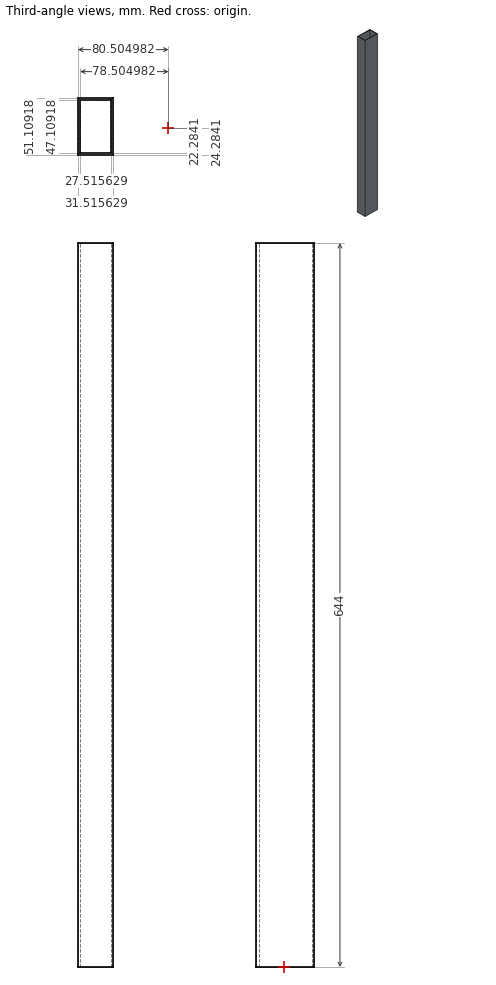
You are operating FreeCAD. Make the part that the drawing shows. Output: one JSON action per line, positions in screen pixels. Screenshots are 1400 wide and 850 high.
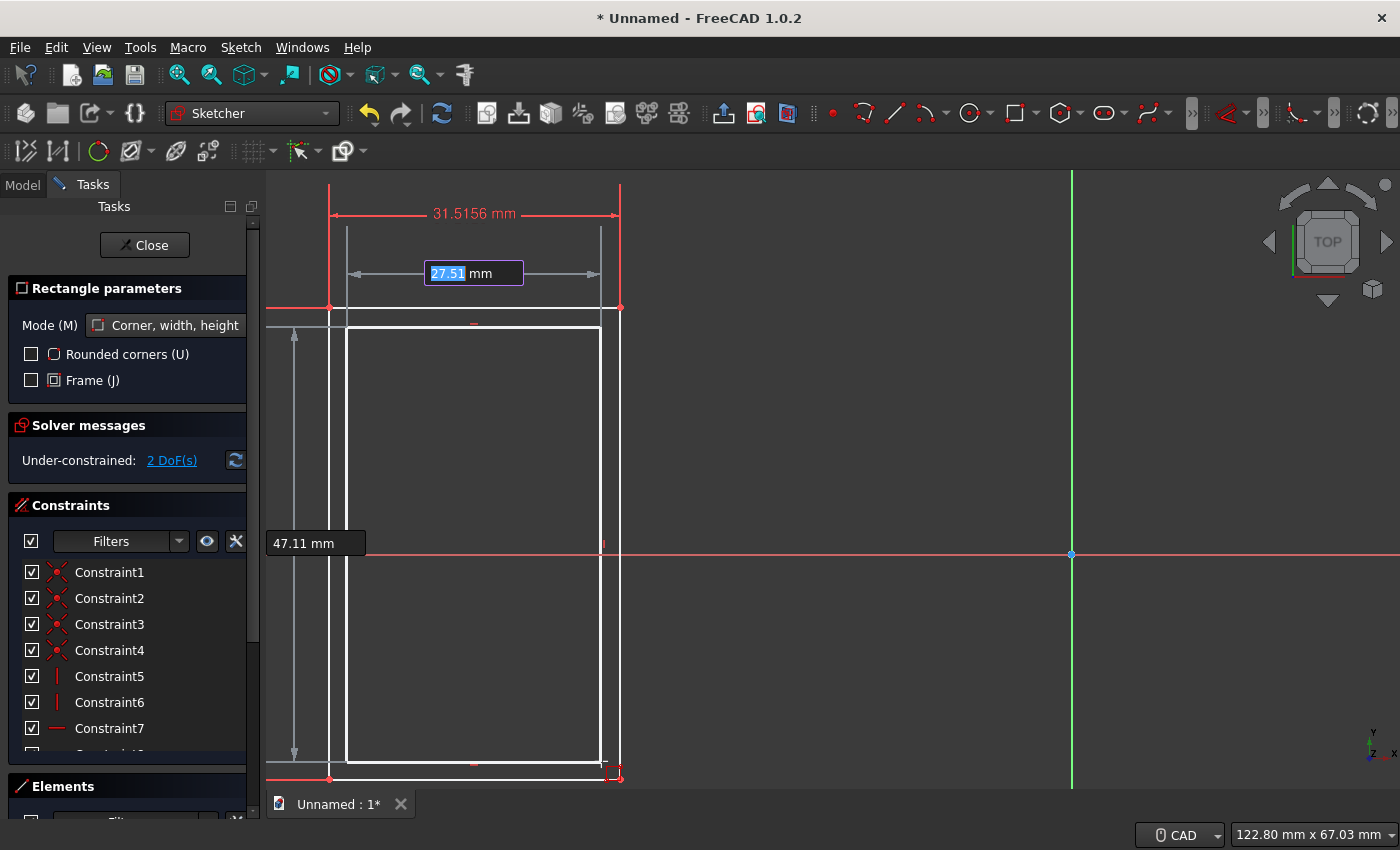
{"action": "type", "text": "27.515629"}
{"action": "key", "text": "Tab"}
{"action": "type", "text": "47.10918"}
{"action": "key", "text": "Return"}
{"action": "key", "text": "Escape"}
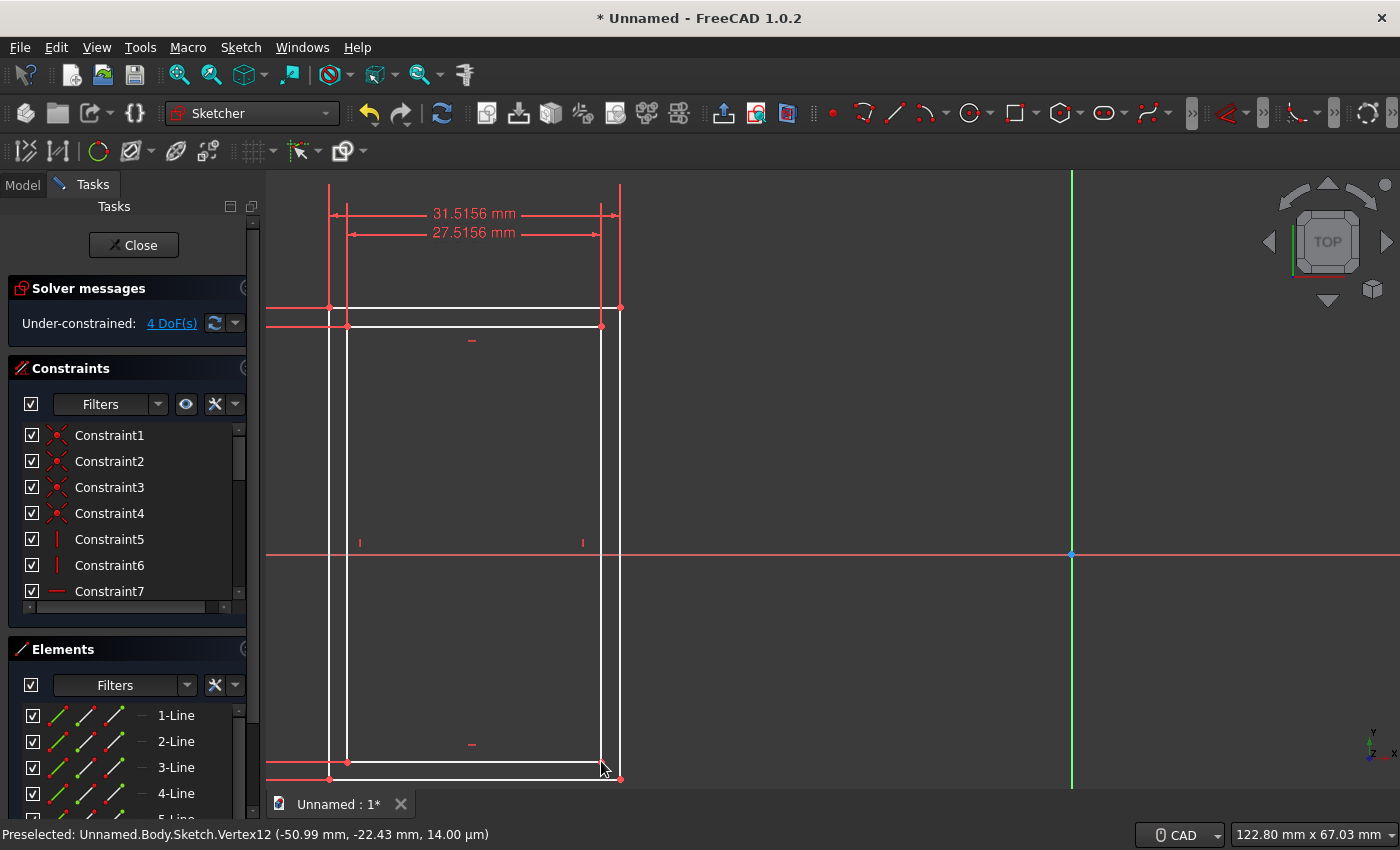
{"action": "left_click", "coordinate": [1226, 114]}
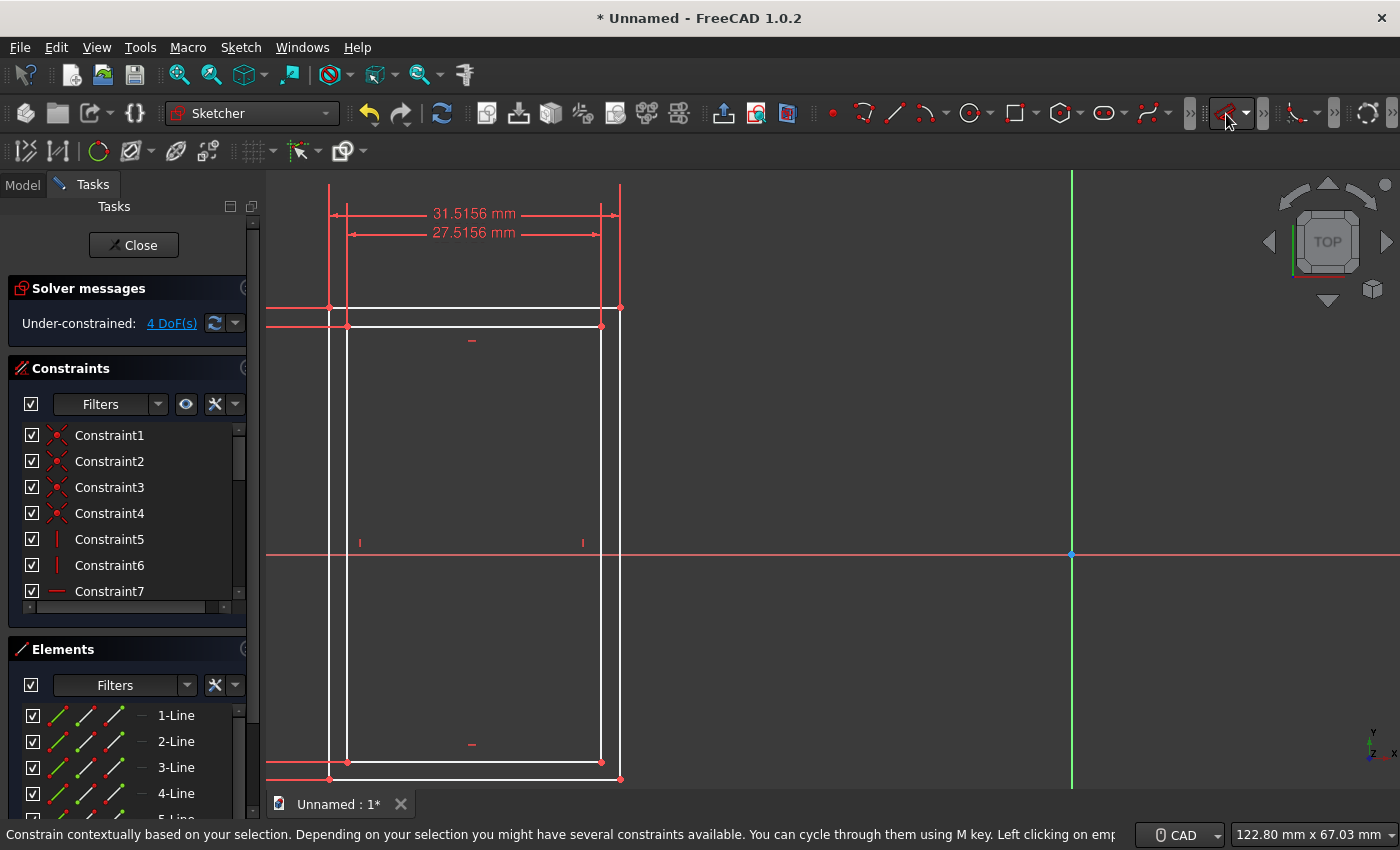
{"action": "scroll", "coordinate": [1055, 198], "scroll_direction": "down", "scroll_amount": 1}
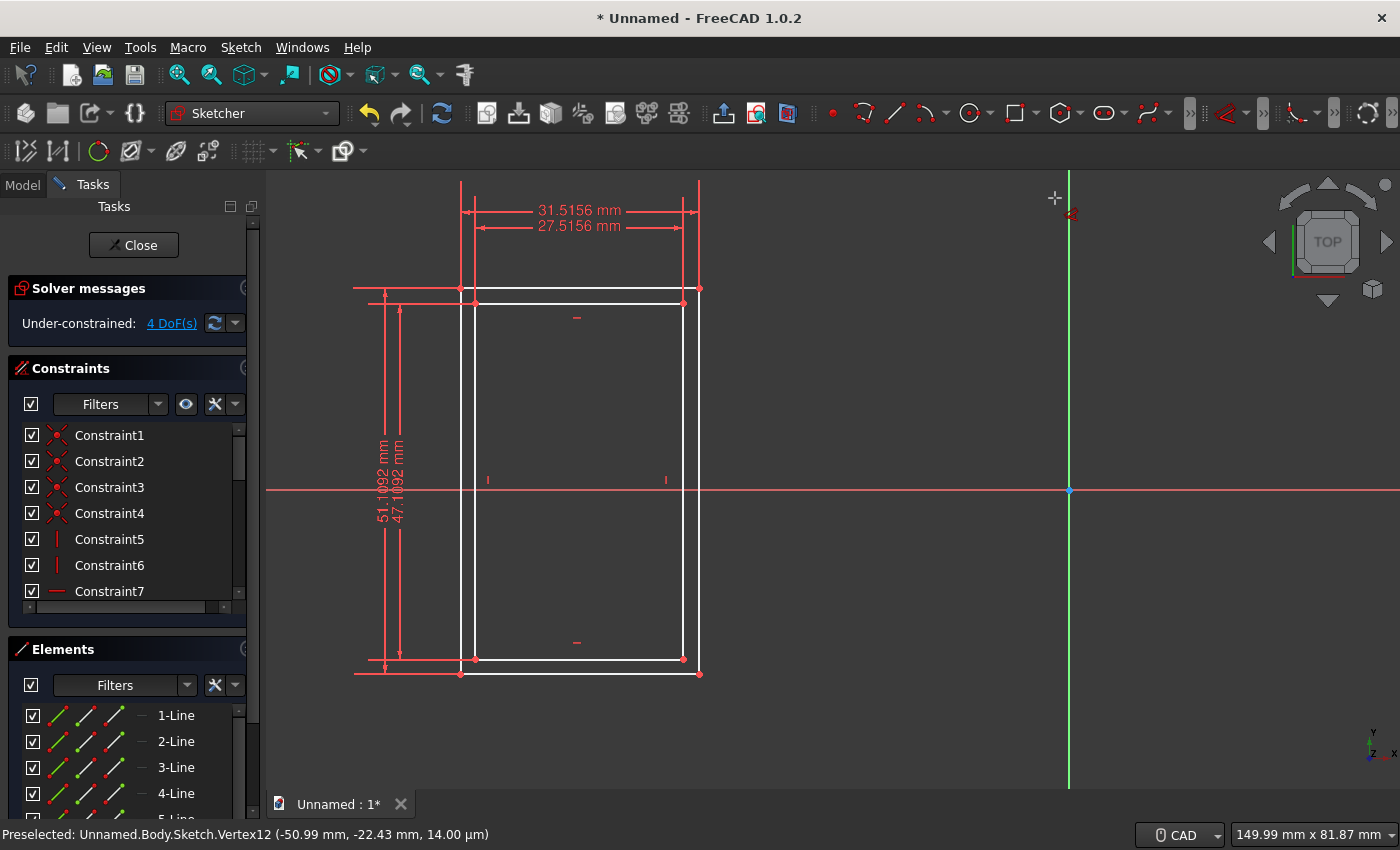
{"action": "left_click", "coordinate": [461, 674]}
{"action": "left_click", "coordinate": [1103, 582]}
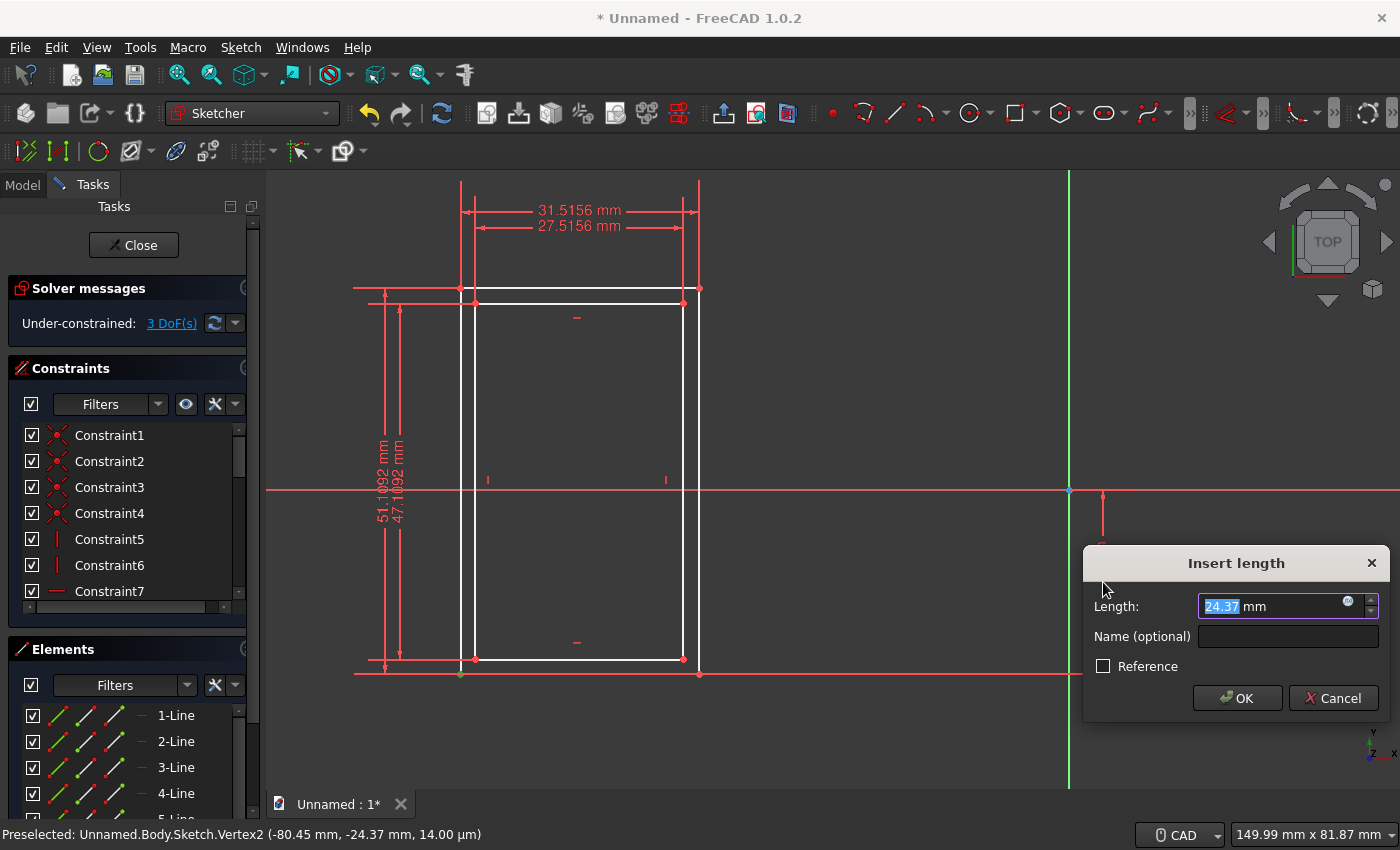
{"action": "type", "text": "24.2841"}
{"action": "key", "text": "Return"}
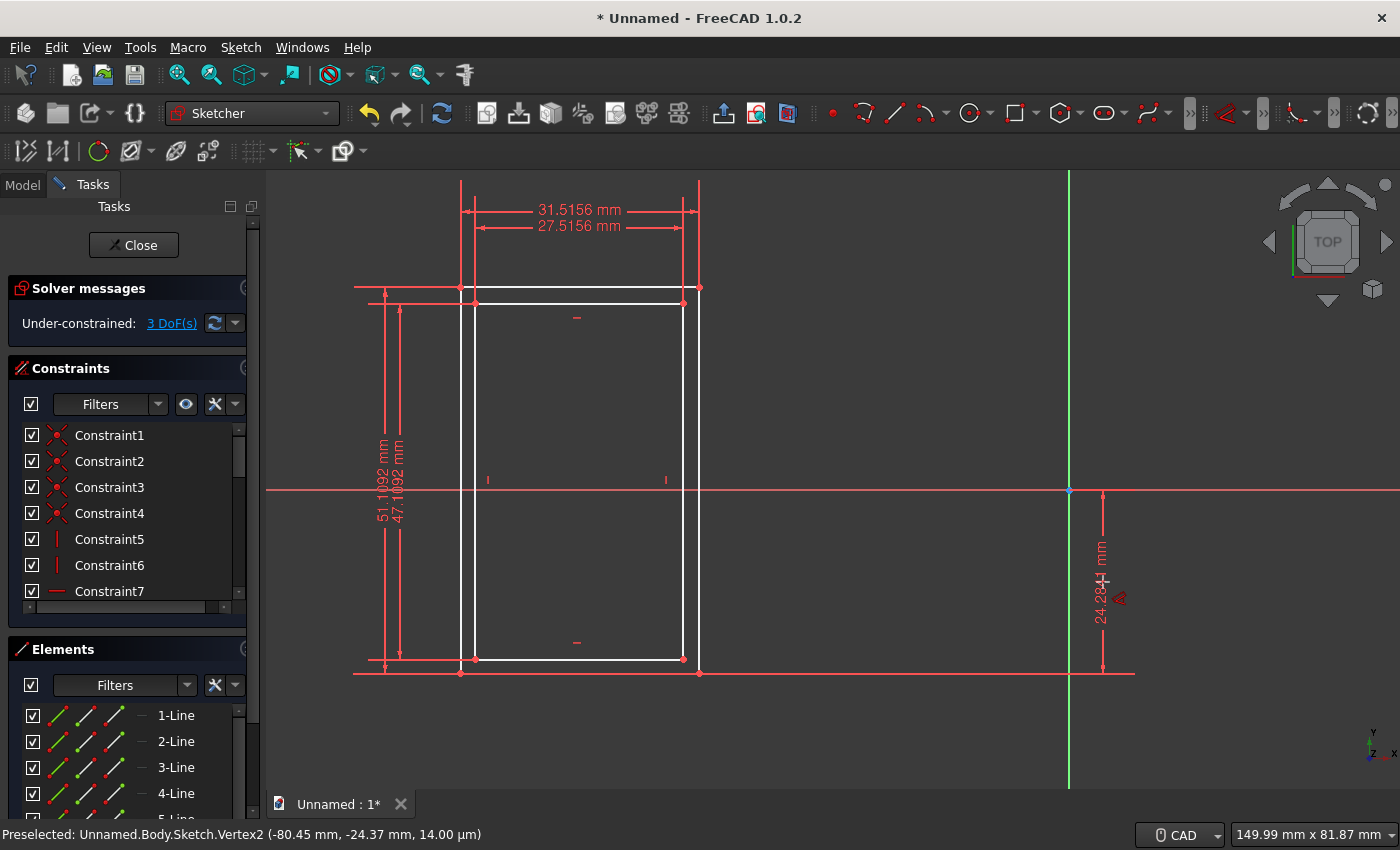
{"action": "left_click", "coordinate": [475, 660]}
{"action": "left_click", "coordinate": [1103, 536]}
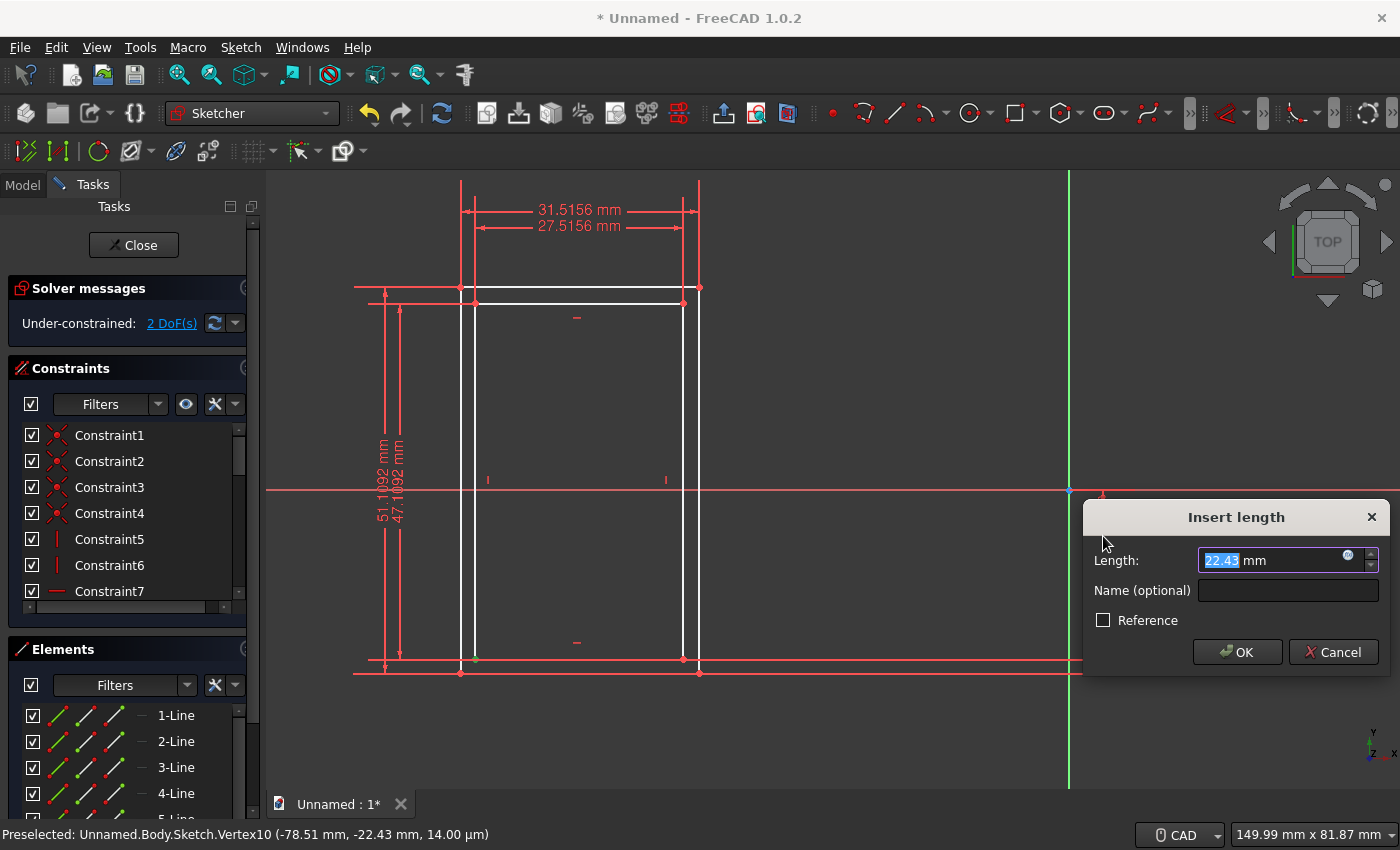
{"action": "type", "text": "22.2841"}
{"action": "key", "text": "Return"}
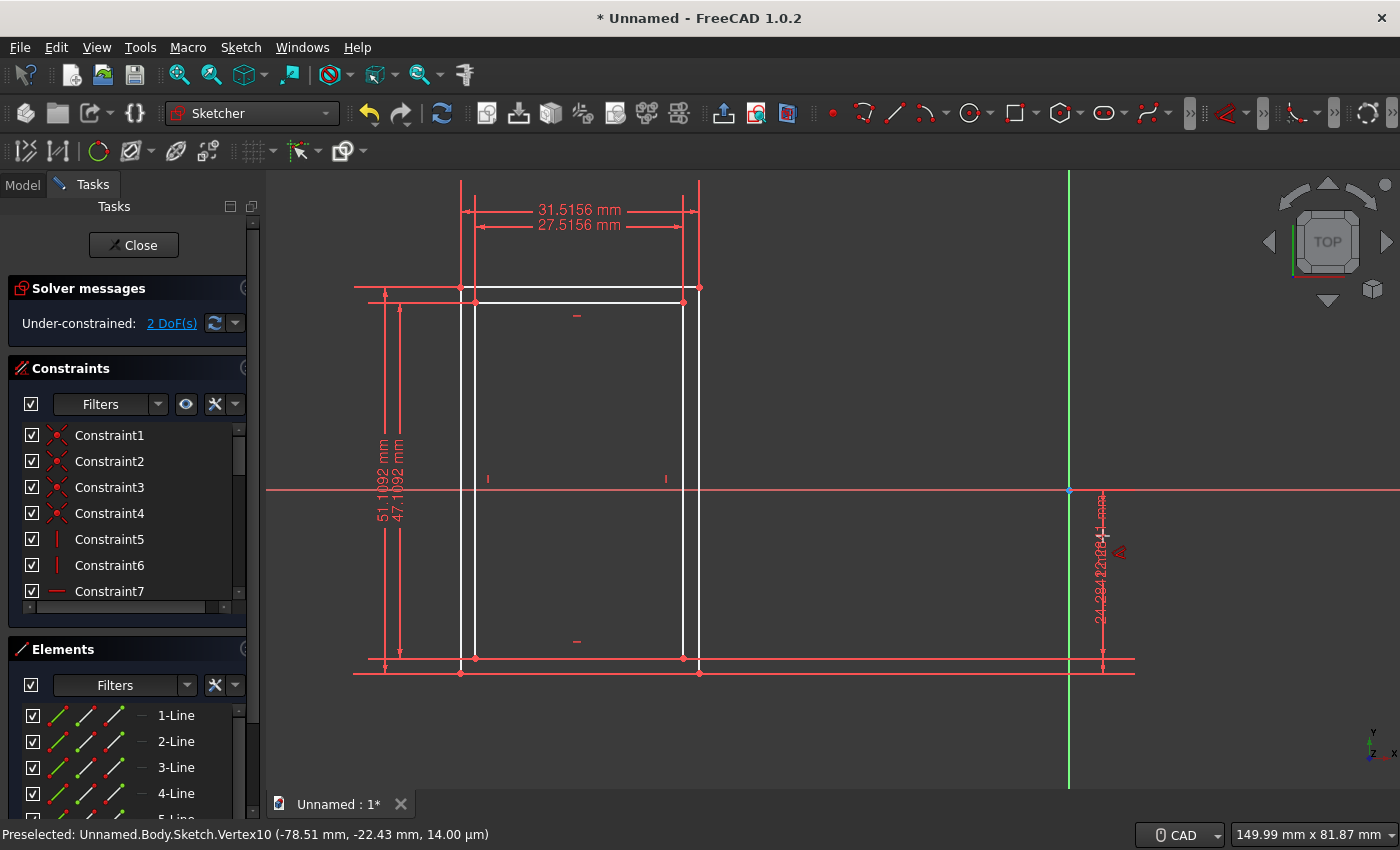
{"action": "left_click", "coordinate": [461, 287]}
{"action": "left_click", "coordinate": [765, 253]}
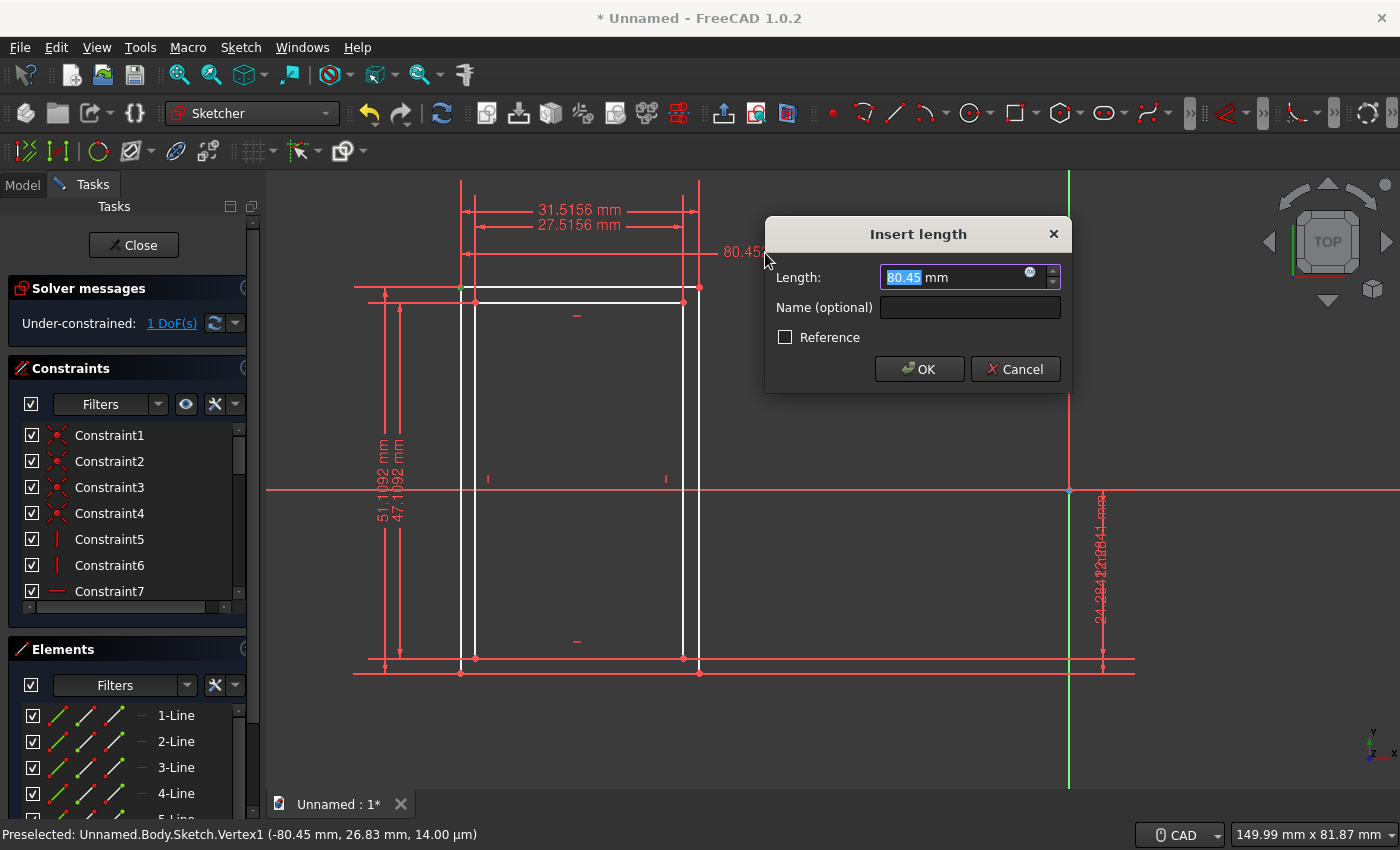
{"action": "type", "text": "80.504982"}
{"action": "key", "text": "Return"}